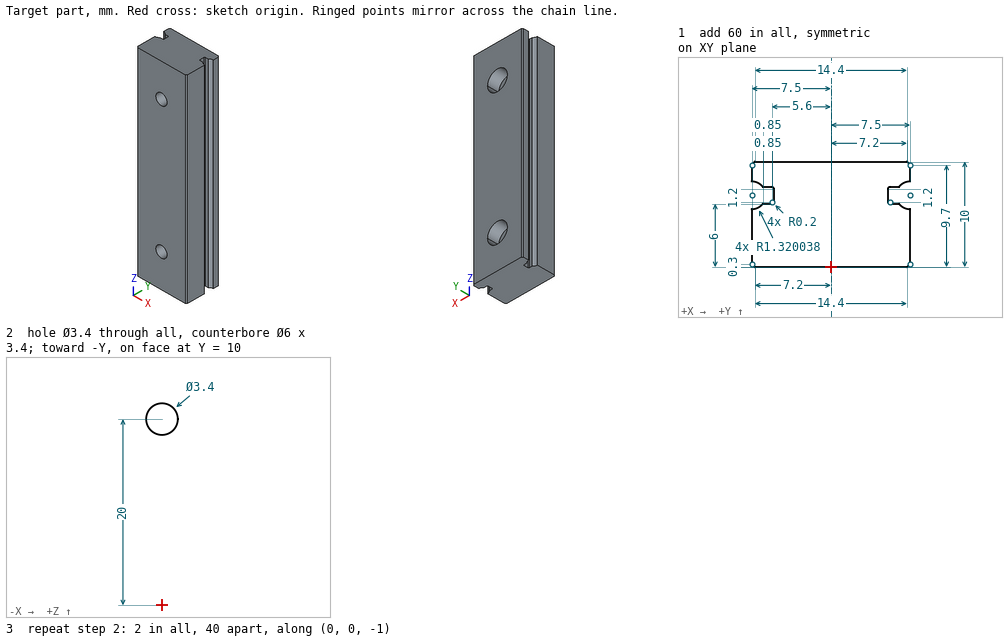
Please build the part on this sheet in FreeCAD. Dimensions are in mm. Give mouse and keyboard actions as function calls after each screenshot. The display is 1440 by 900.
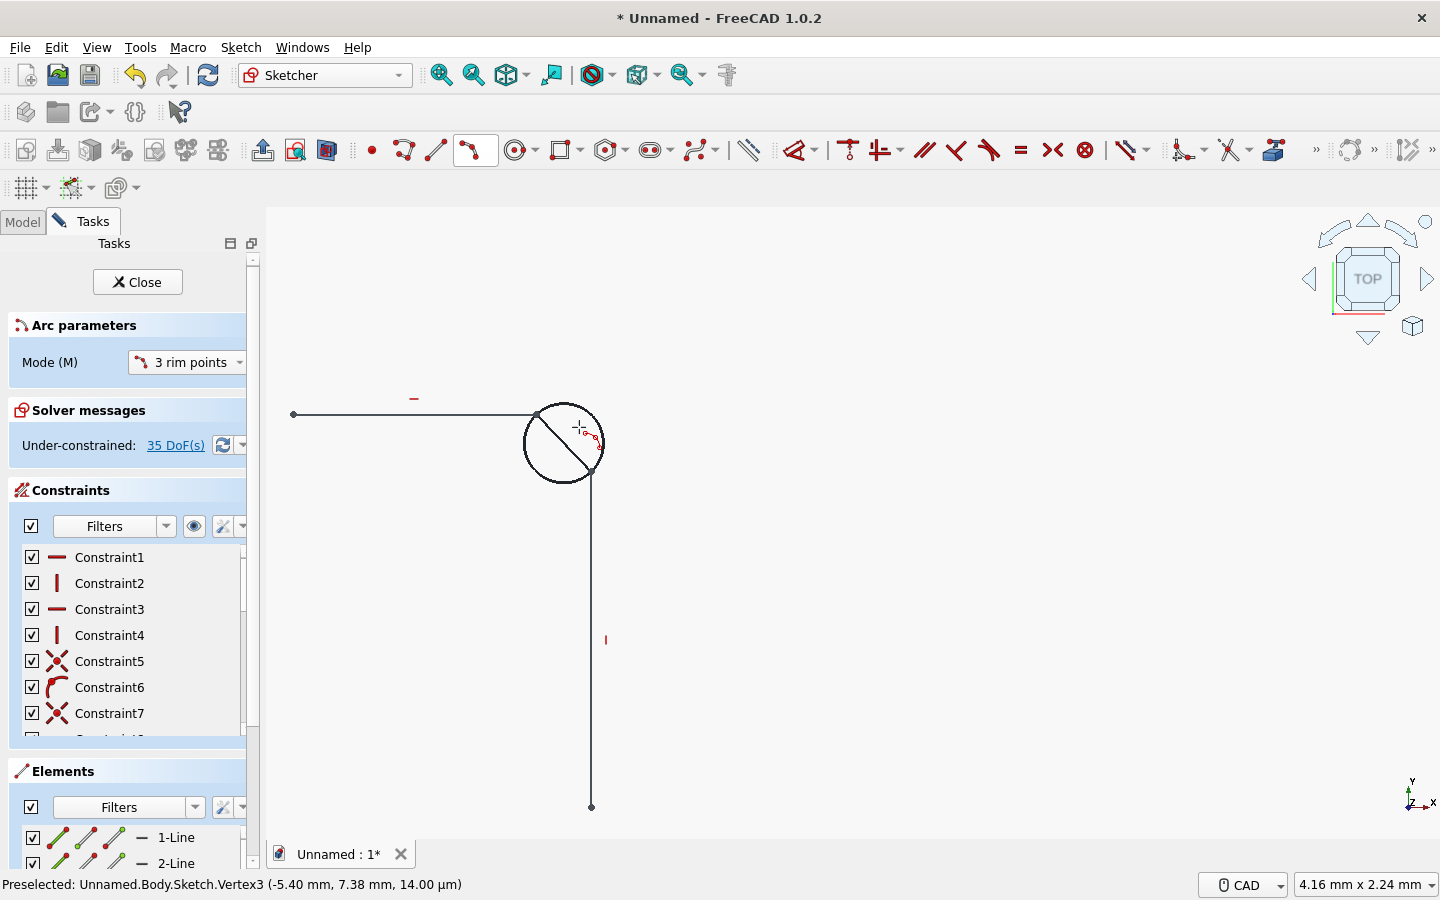
click(576, 425)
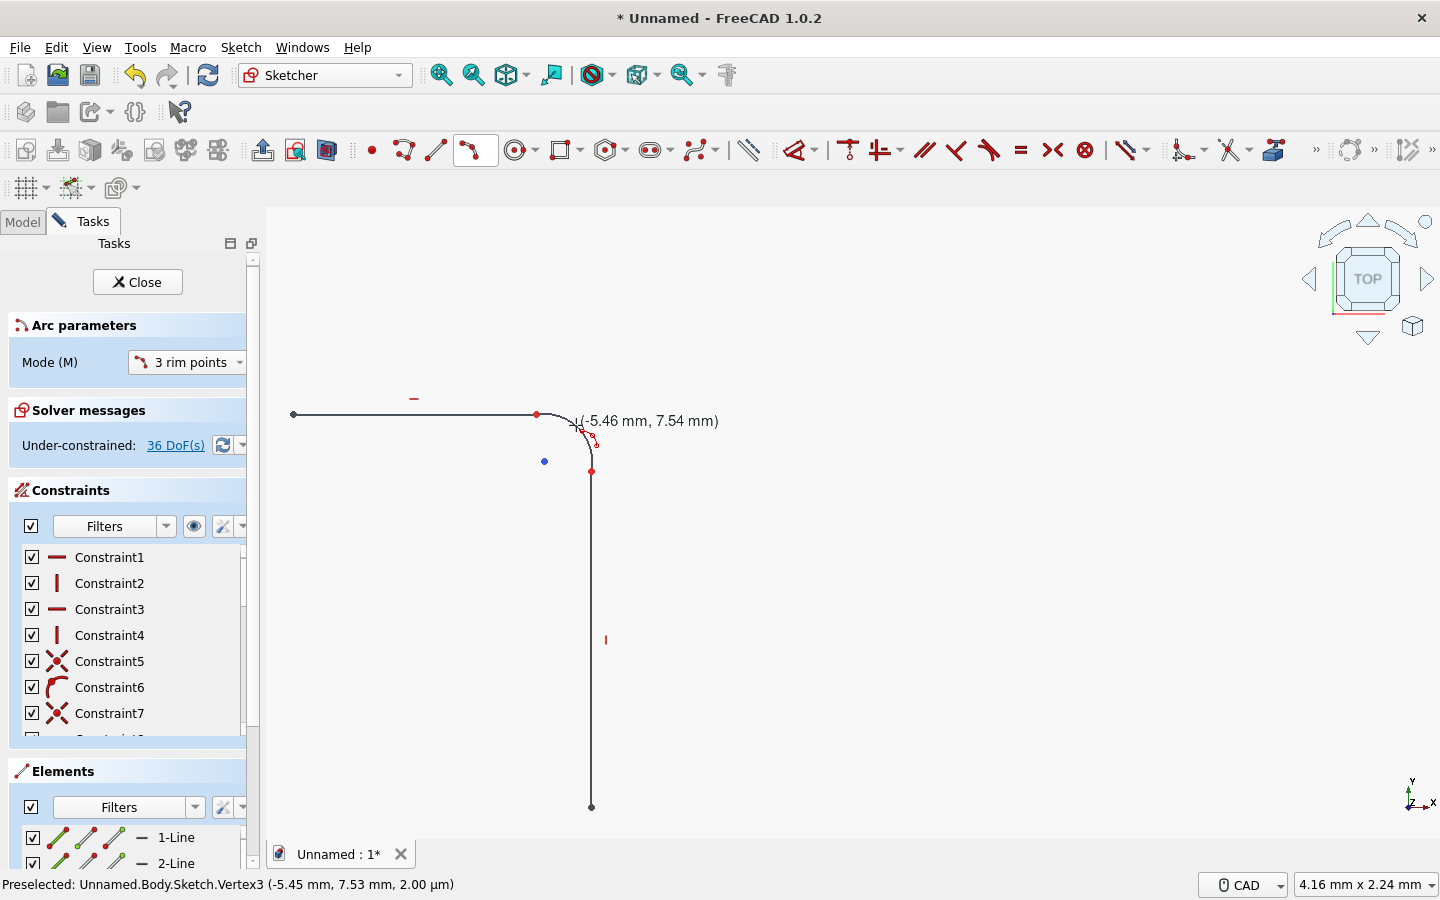
scroll(576, 426, down, 10)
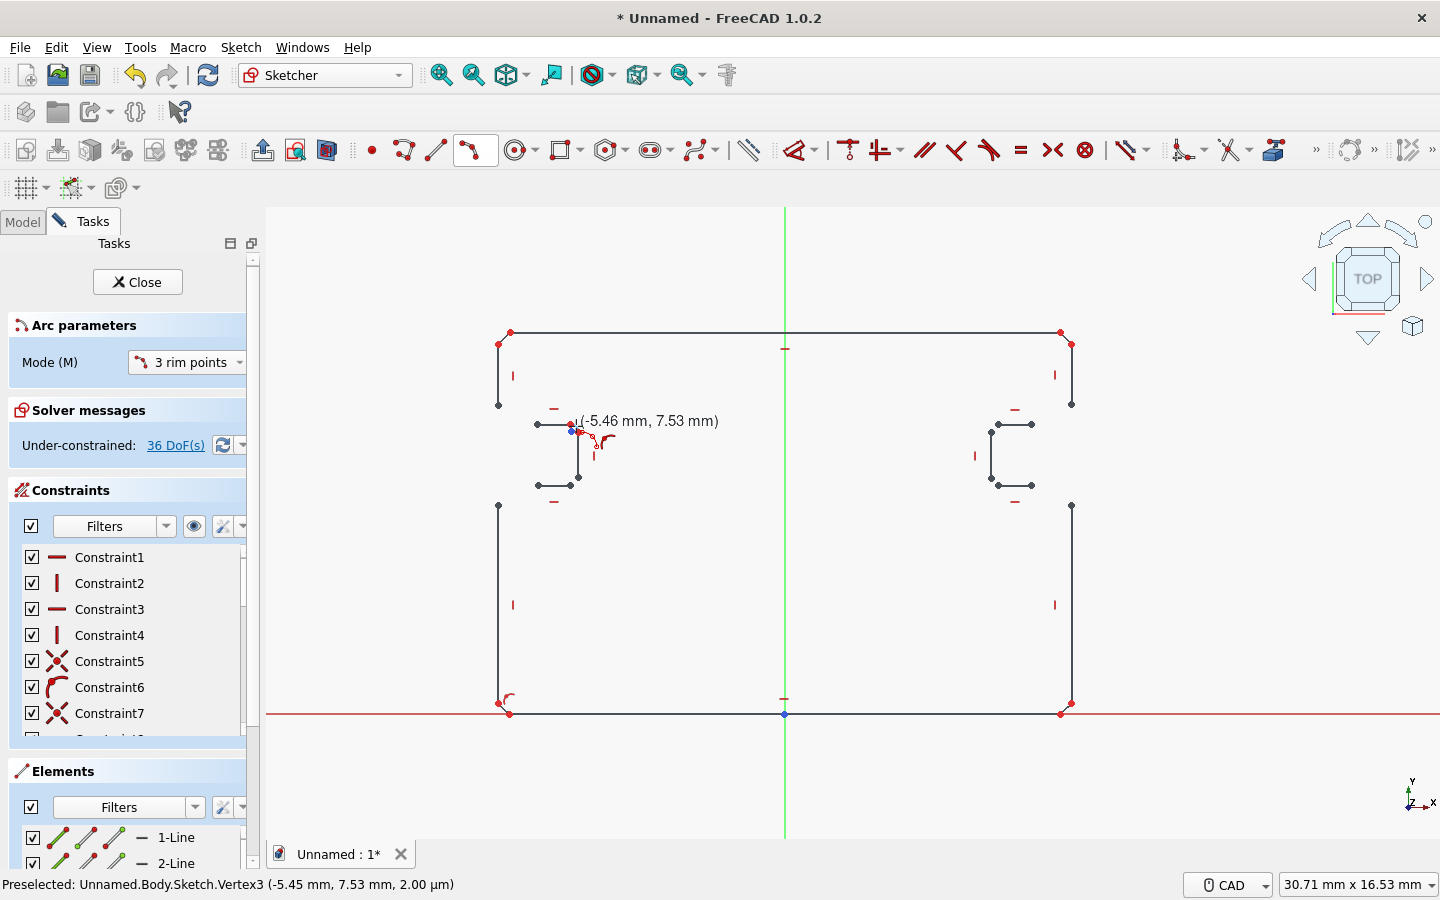
scroll(578, 477, up, 2)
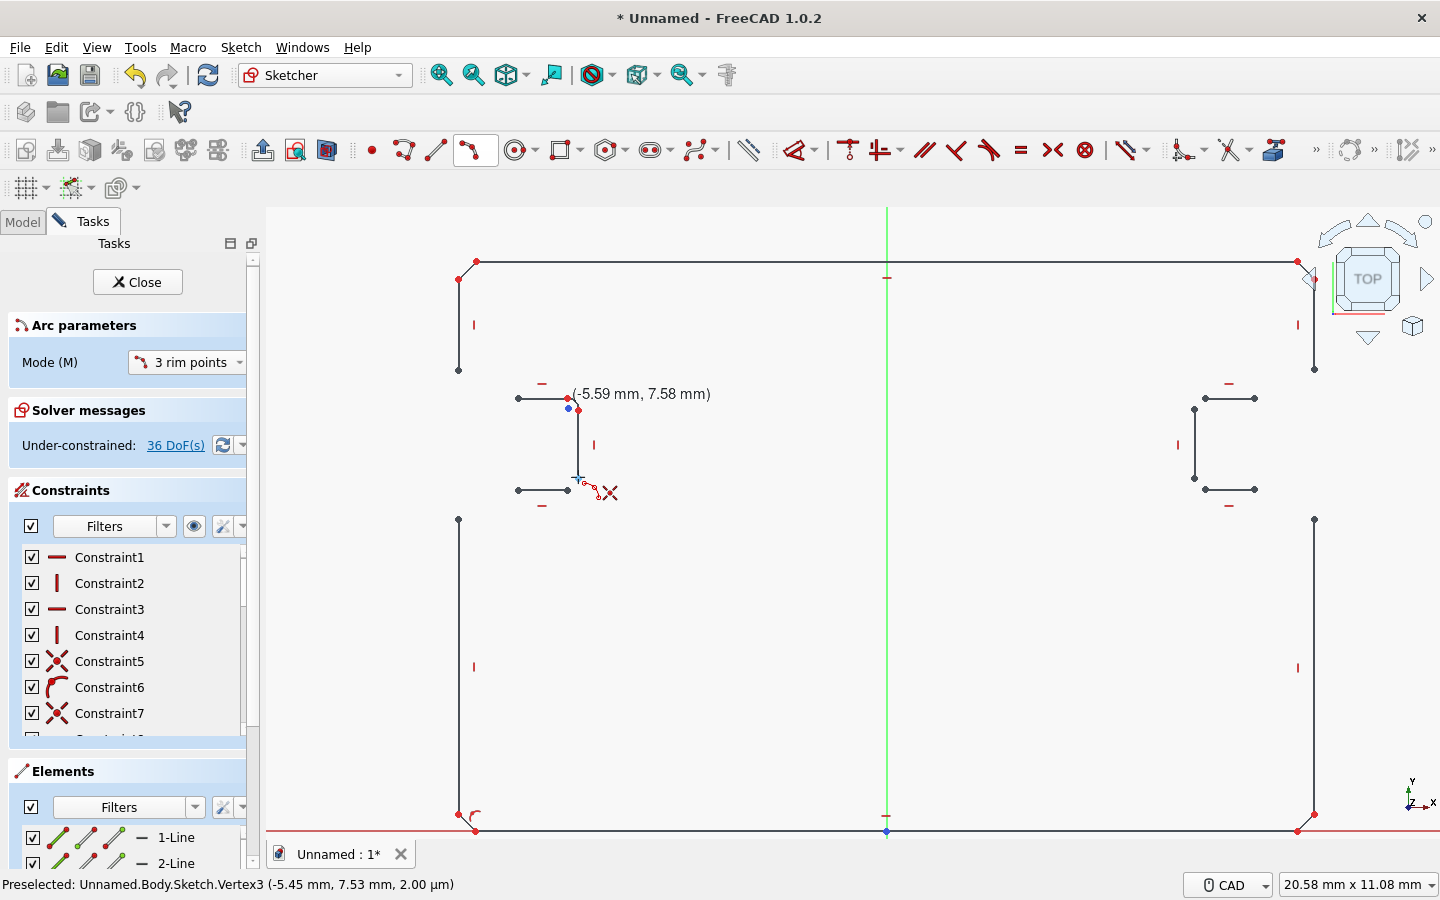
click(578, 478)
click(567, 490)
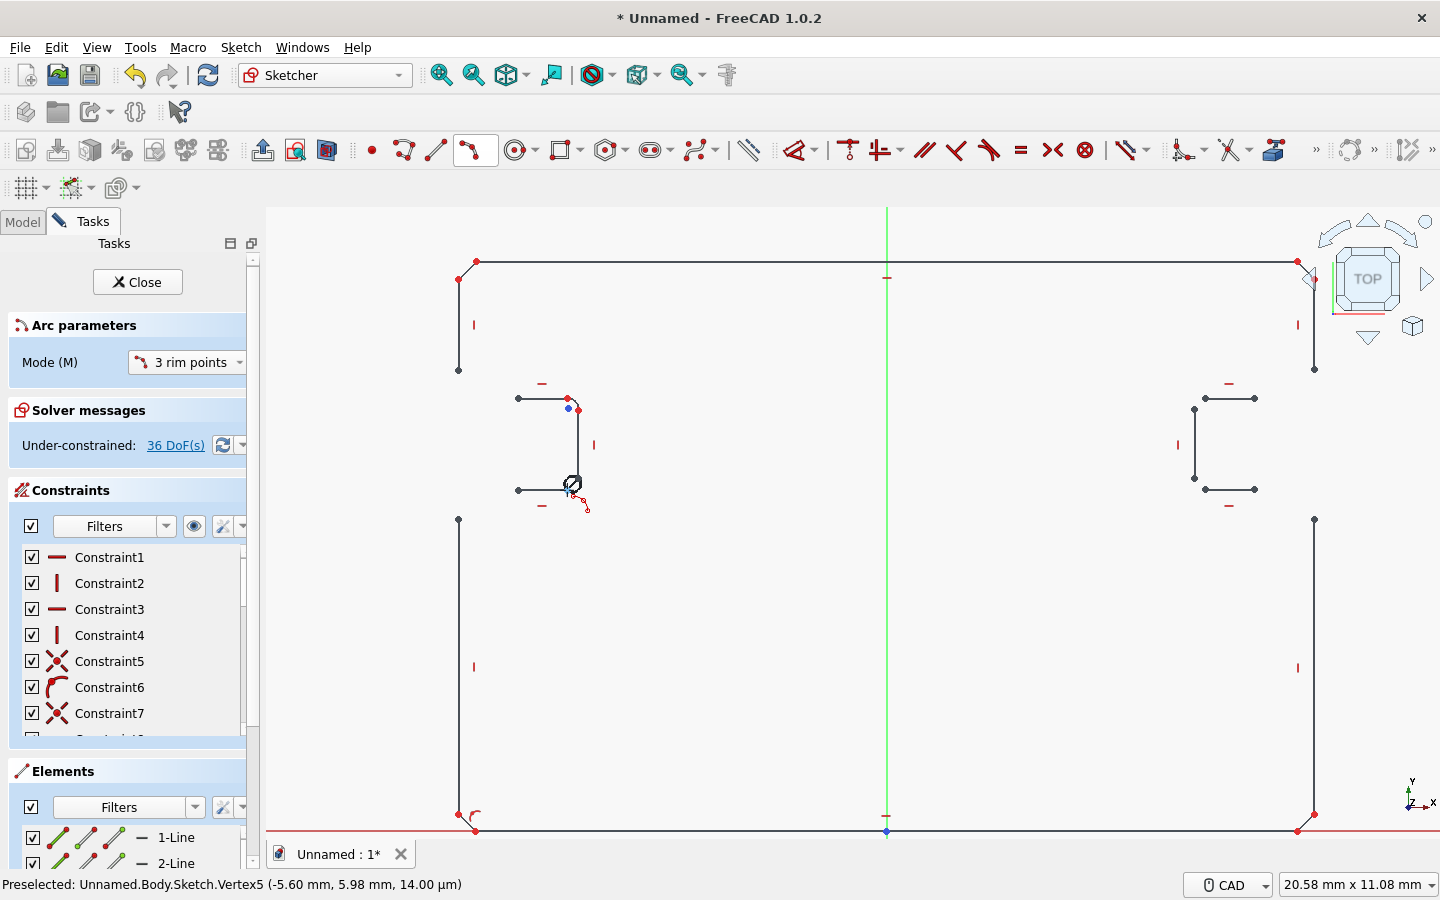
scroll(575, 486, up, 8)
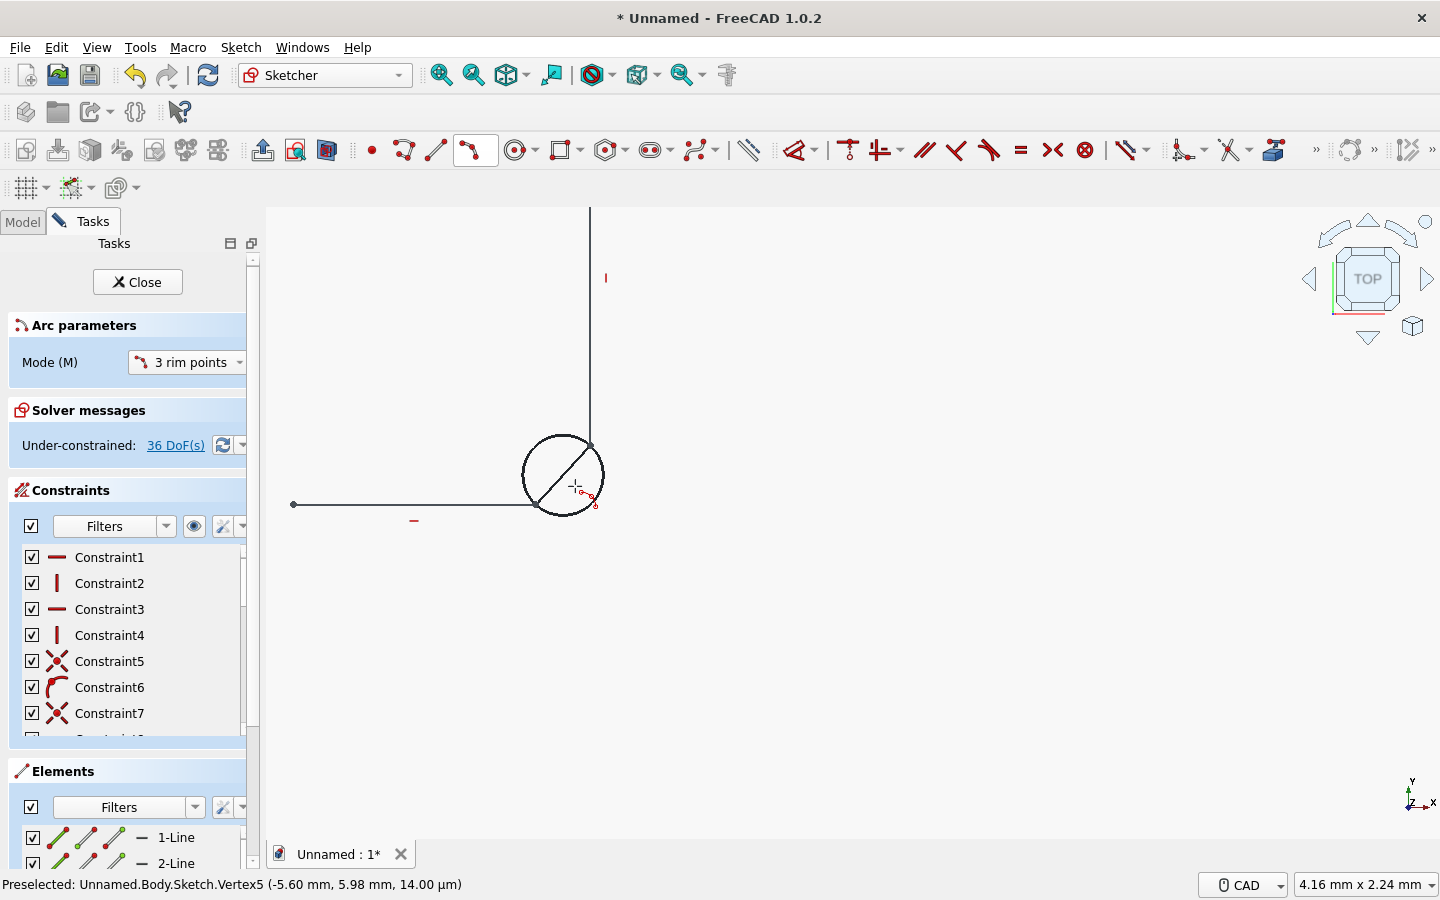
click(575, 482)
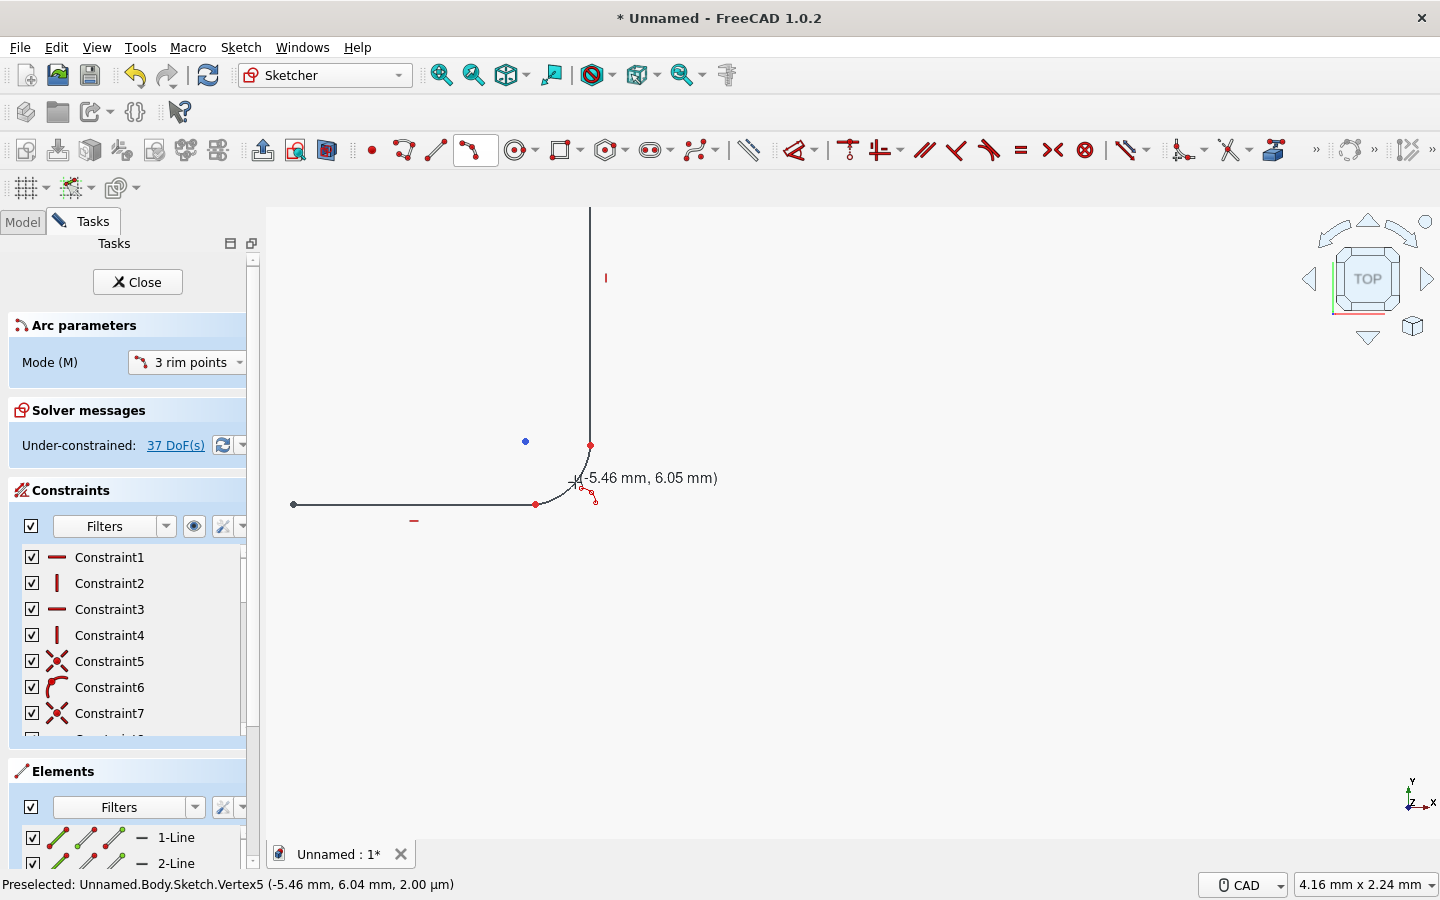
scroll(576, 483, down, 10)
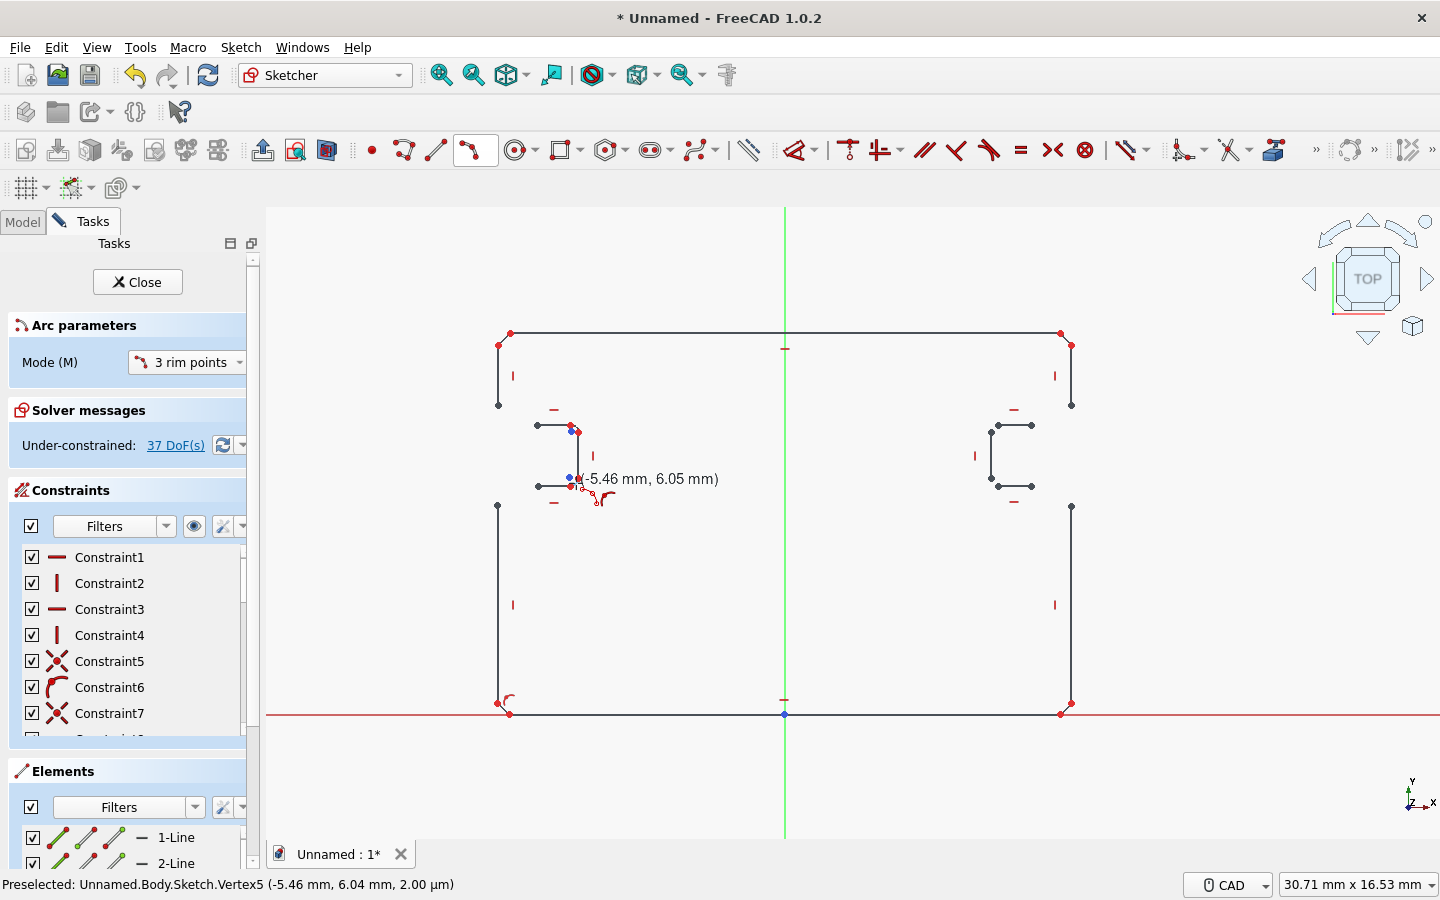
click(538, 486)
click(498, 506)